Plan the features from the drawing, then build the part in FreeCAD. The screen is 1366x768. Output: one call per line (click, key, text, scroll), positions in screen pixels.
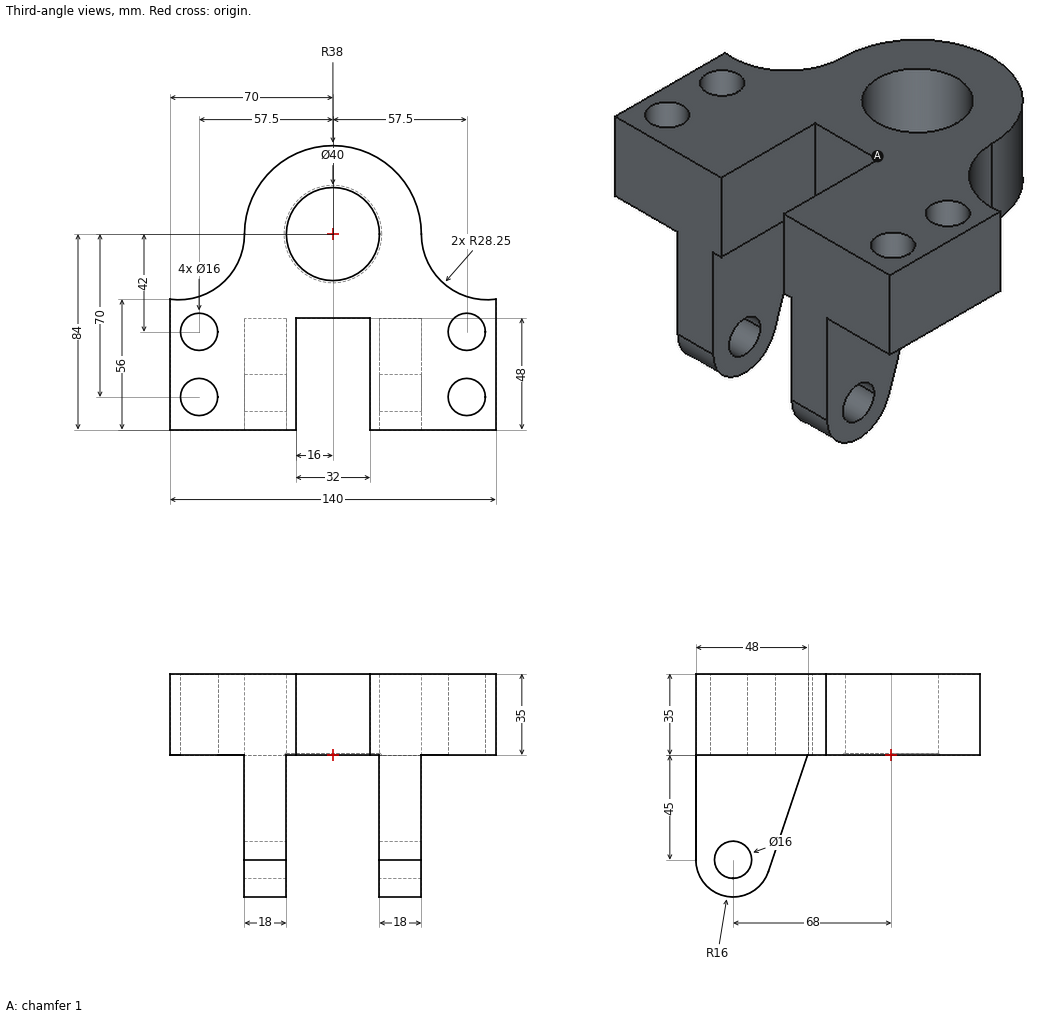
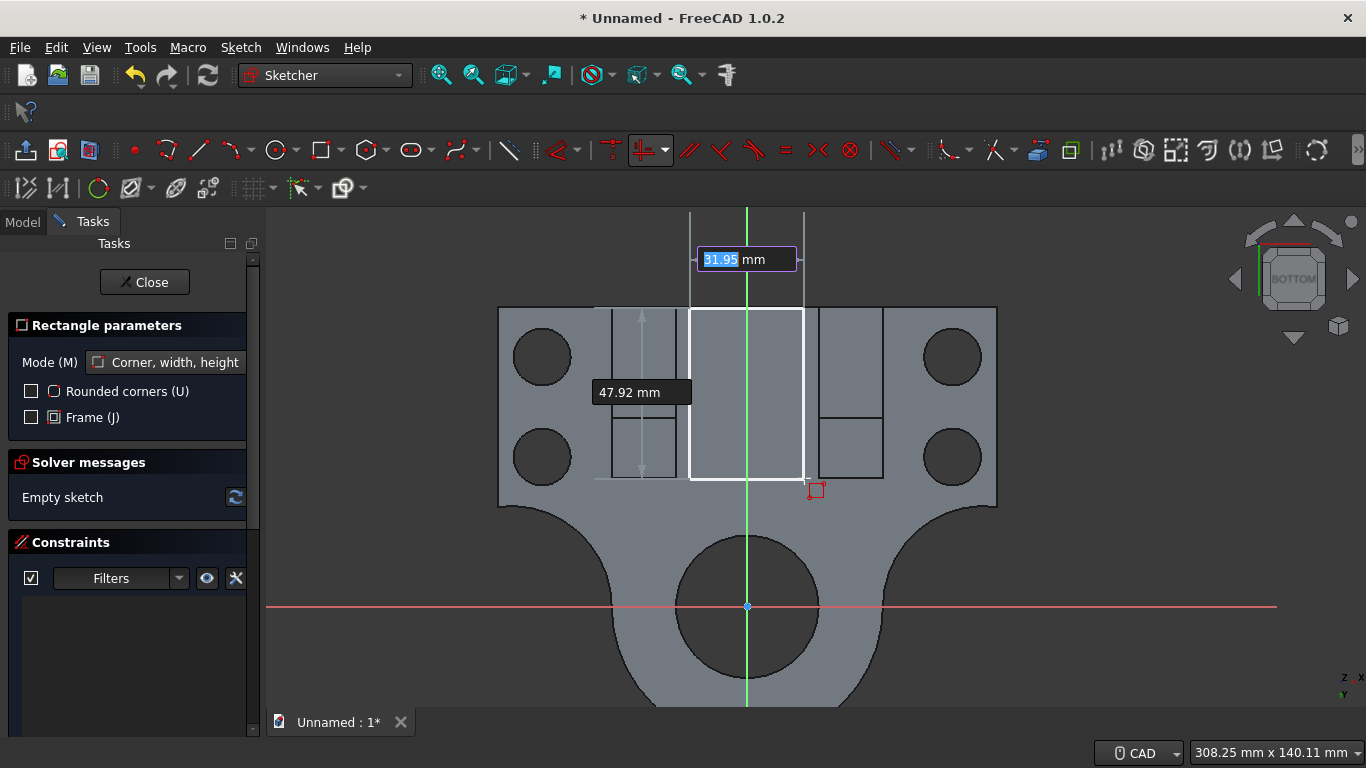
text(32)
key(Tab)
text(48)
key(Return)
key(Escape)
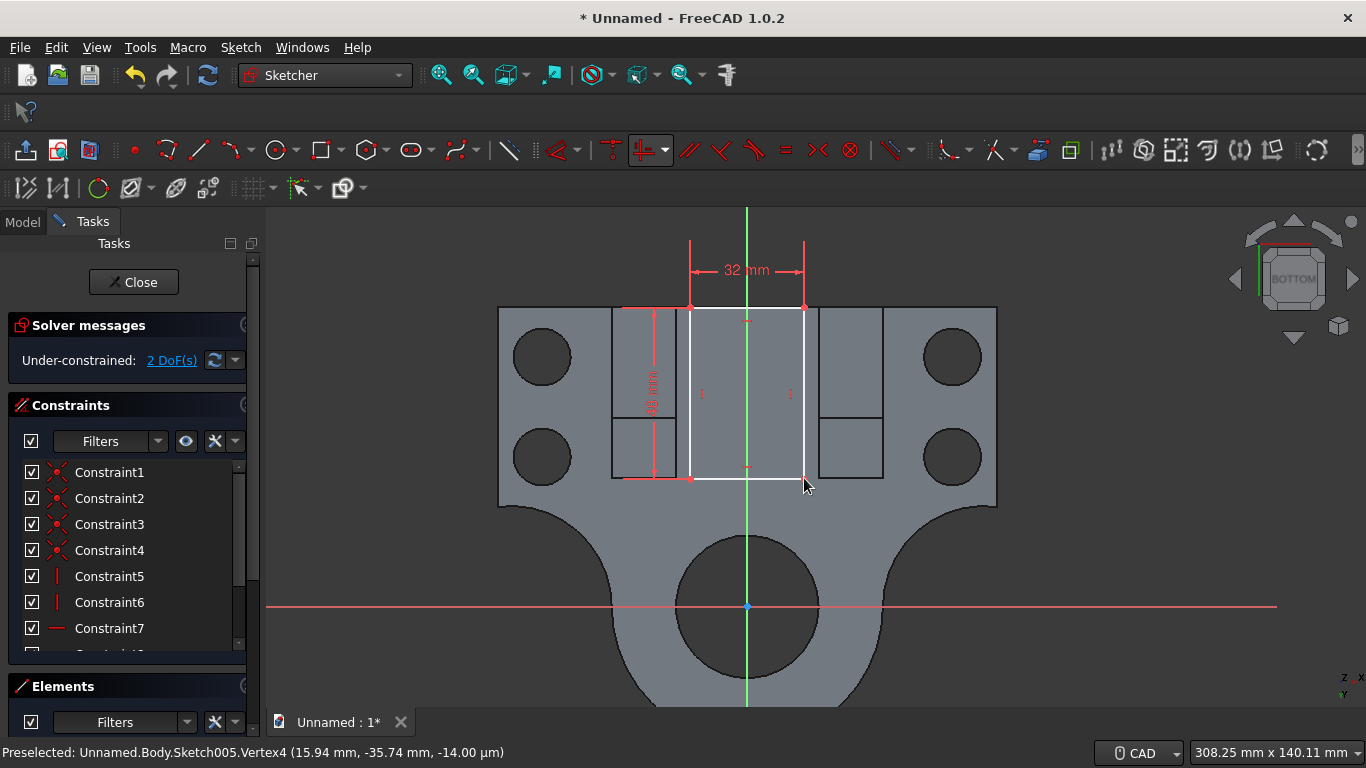
click(556, 150)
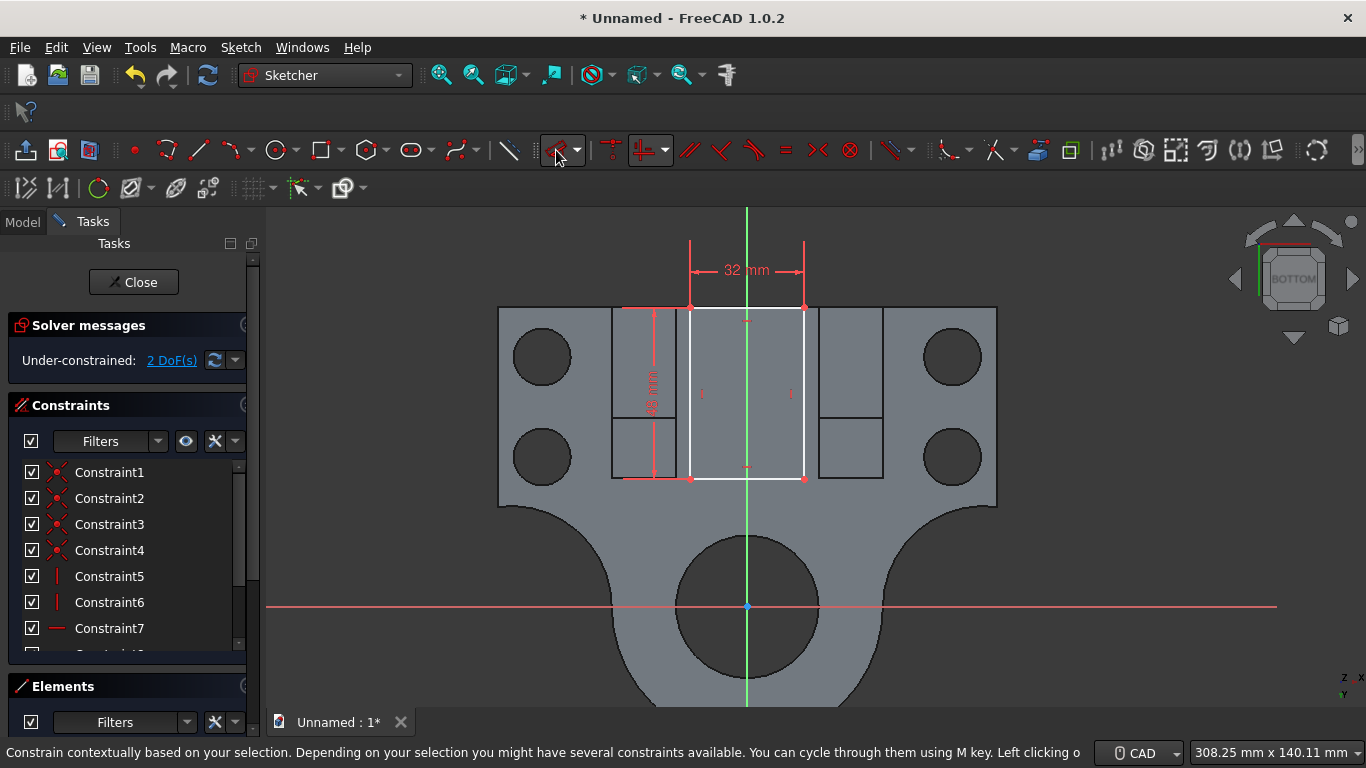
click(690, 308)
click(719, 641)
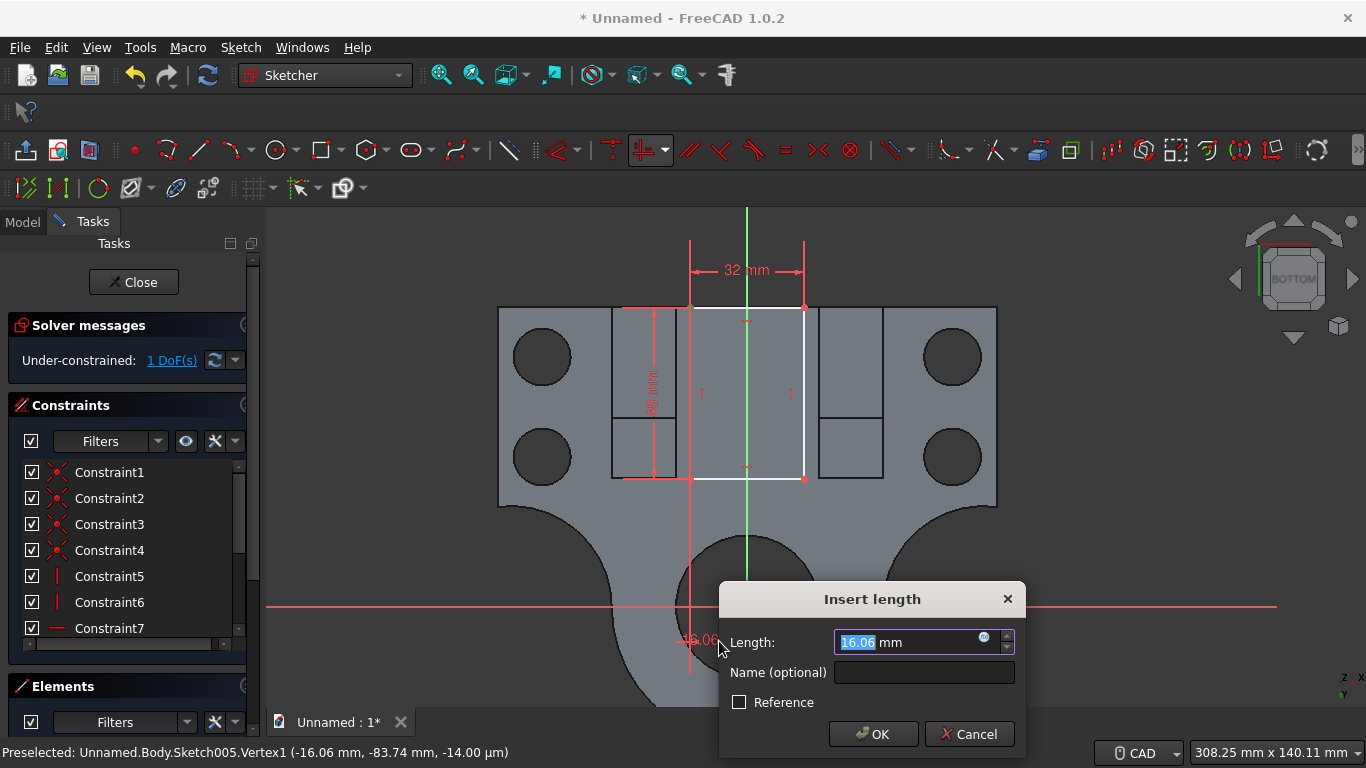
text(16)
key(Return)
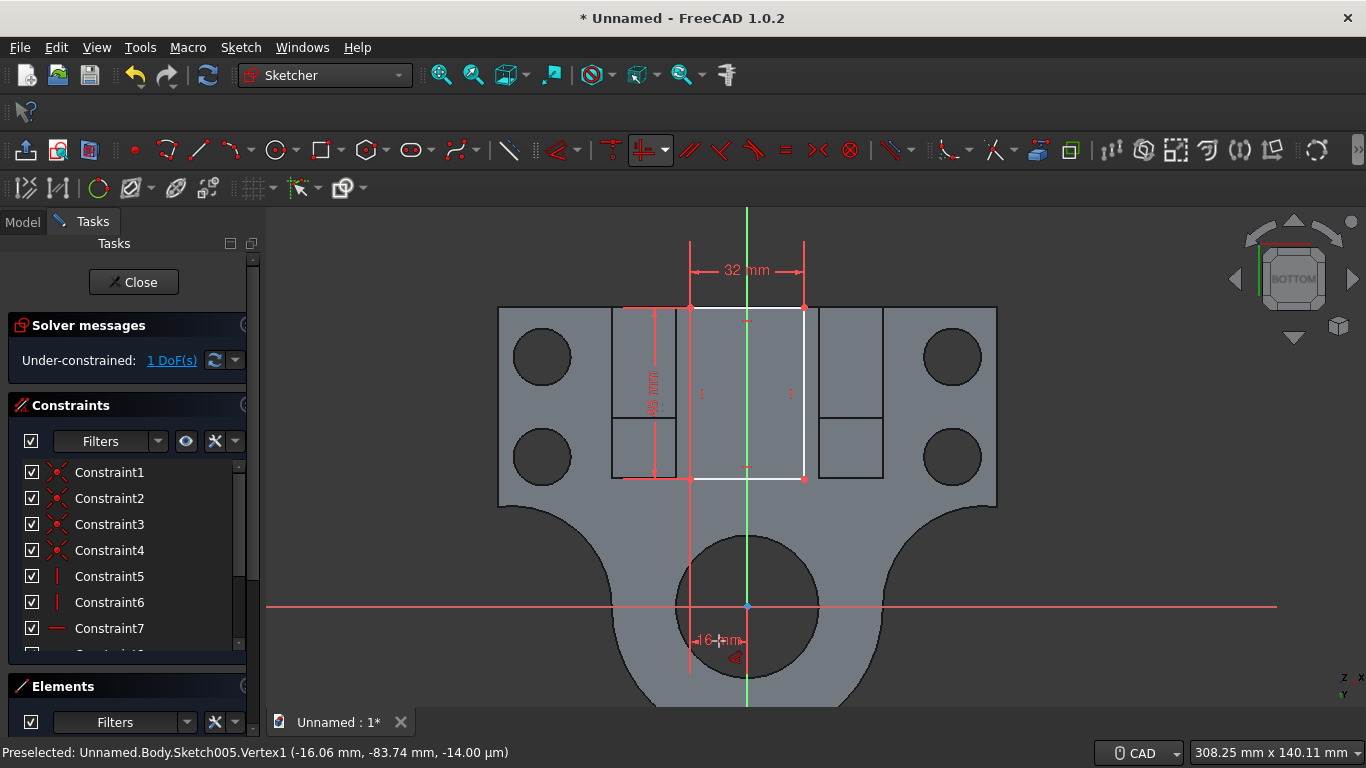
click(690, 308)
click(656, 457)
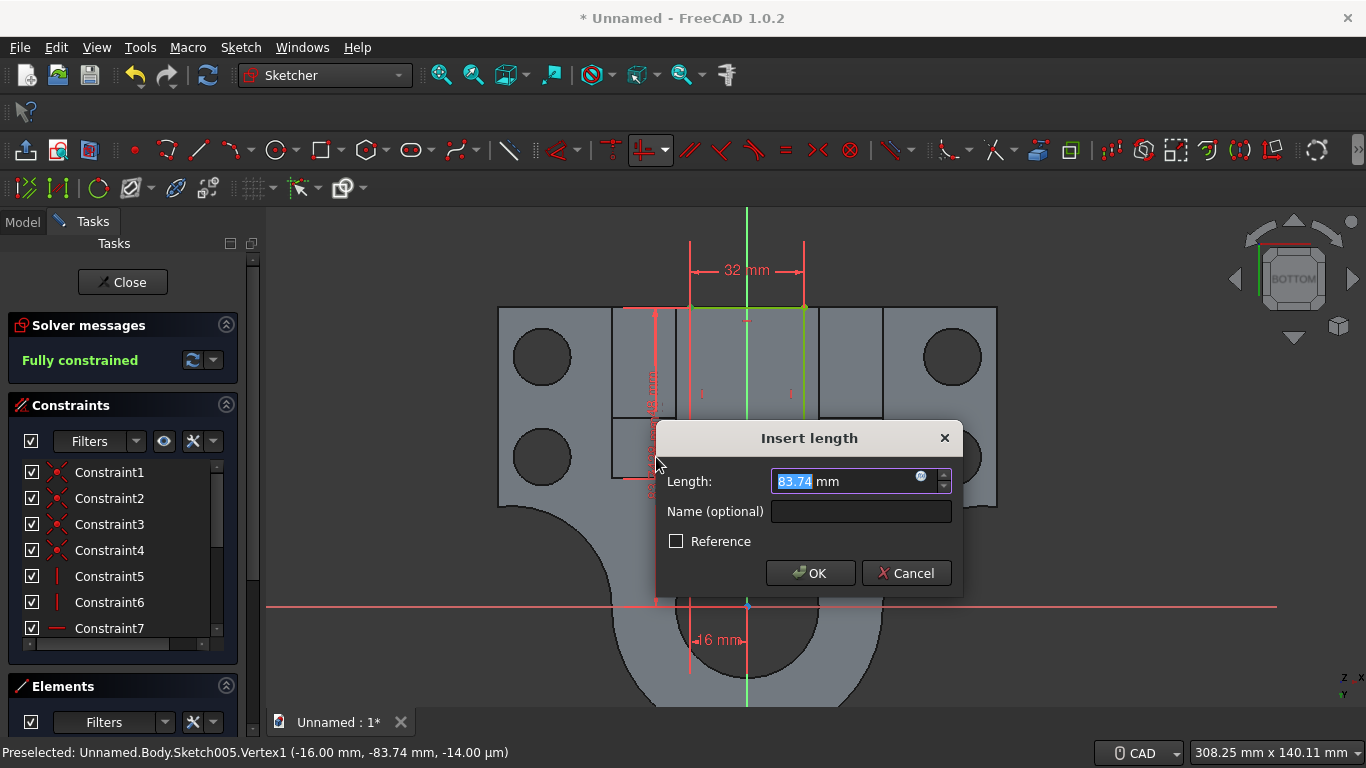
text(84)
key(Return)
key(Escape)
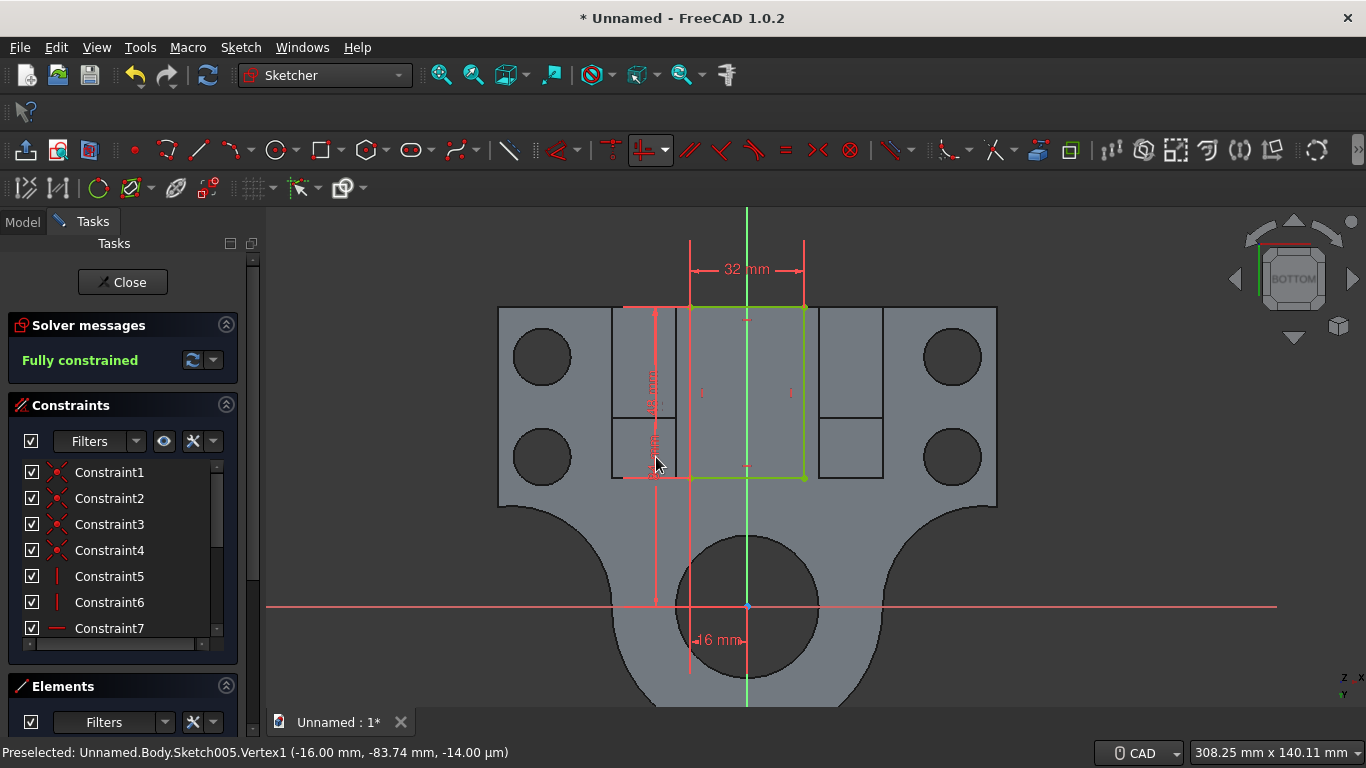
click(123, 282)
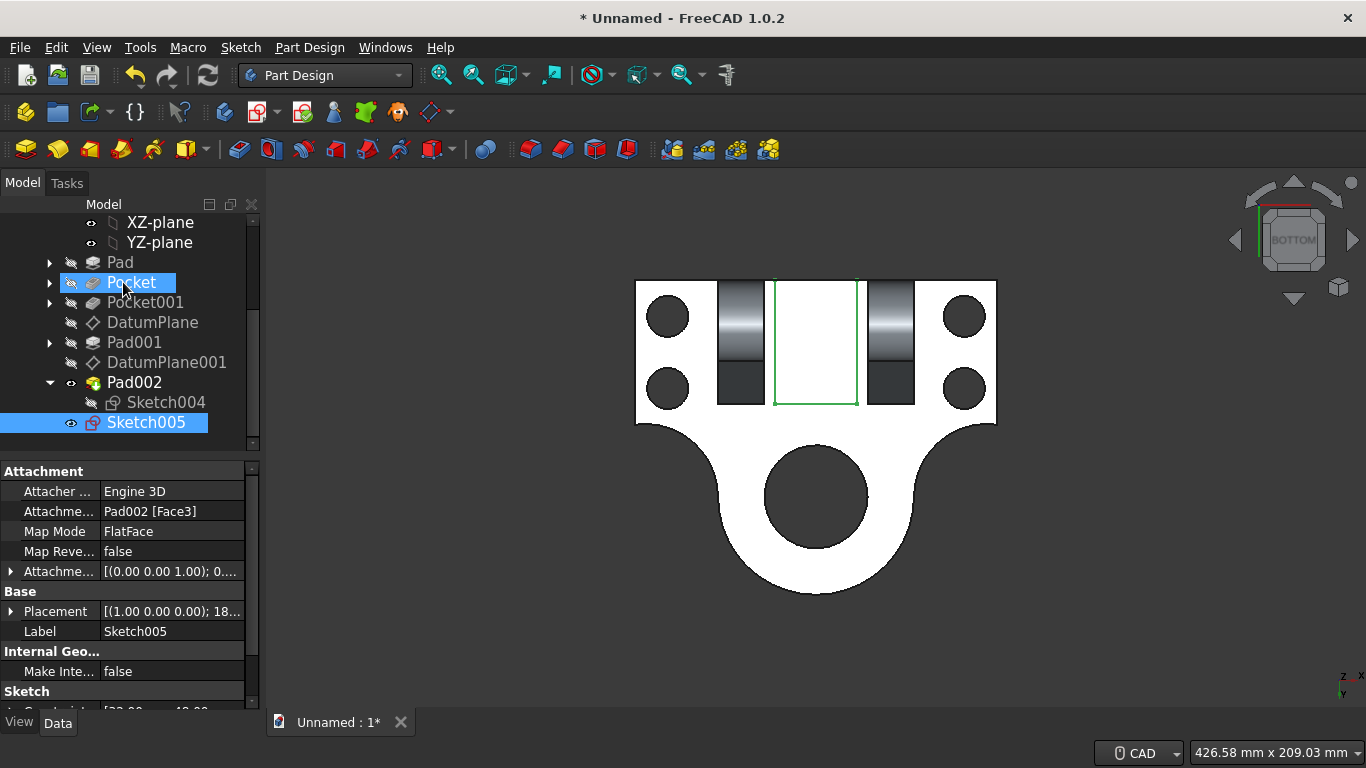
click(240, 150)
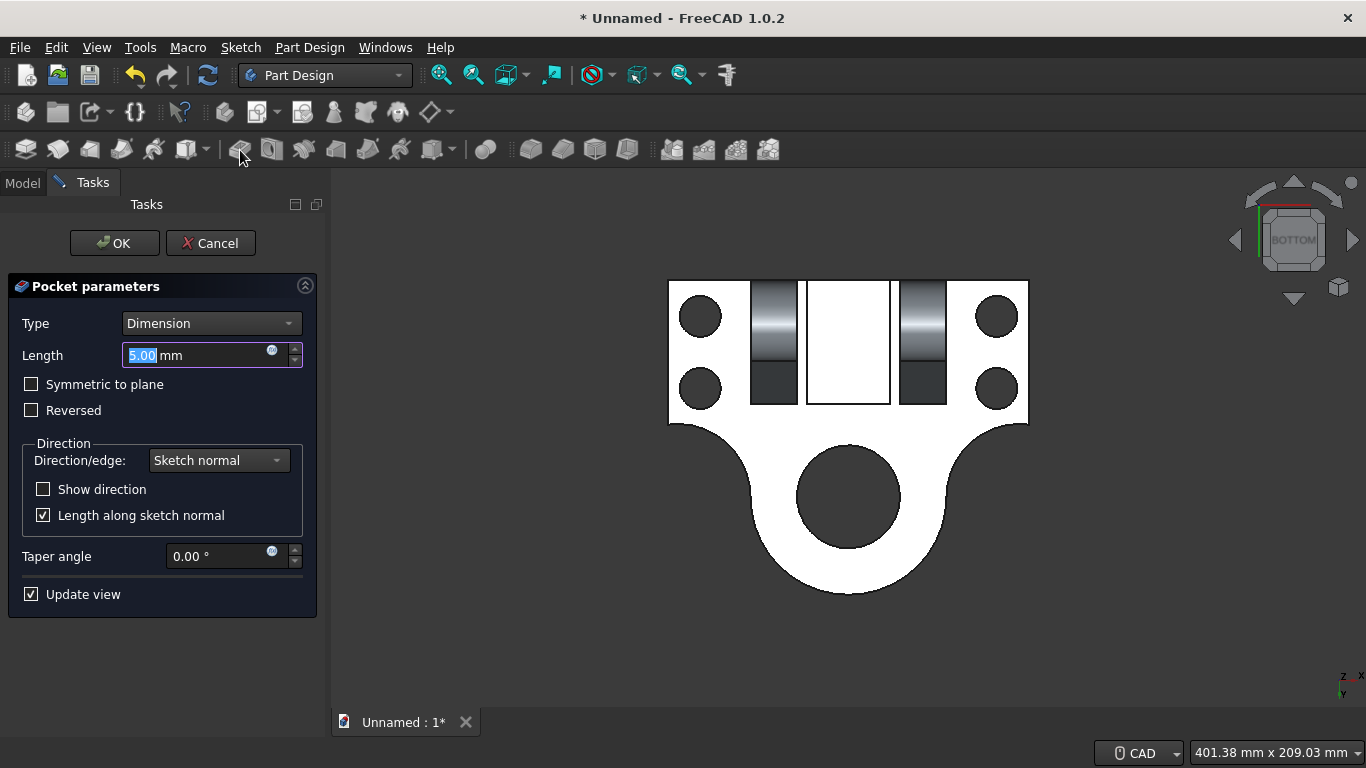
text(35)
key(Tab)